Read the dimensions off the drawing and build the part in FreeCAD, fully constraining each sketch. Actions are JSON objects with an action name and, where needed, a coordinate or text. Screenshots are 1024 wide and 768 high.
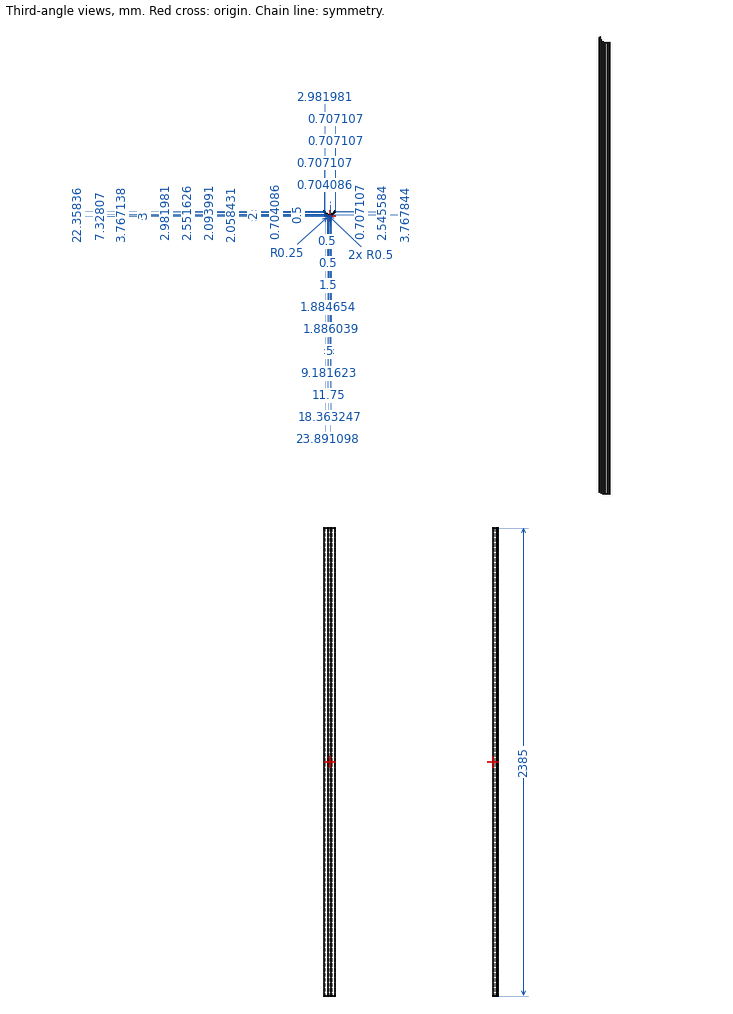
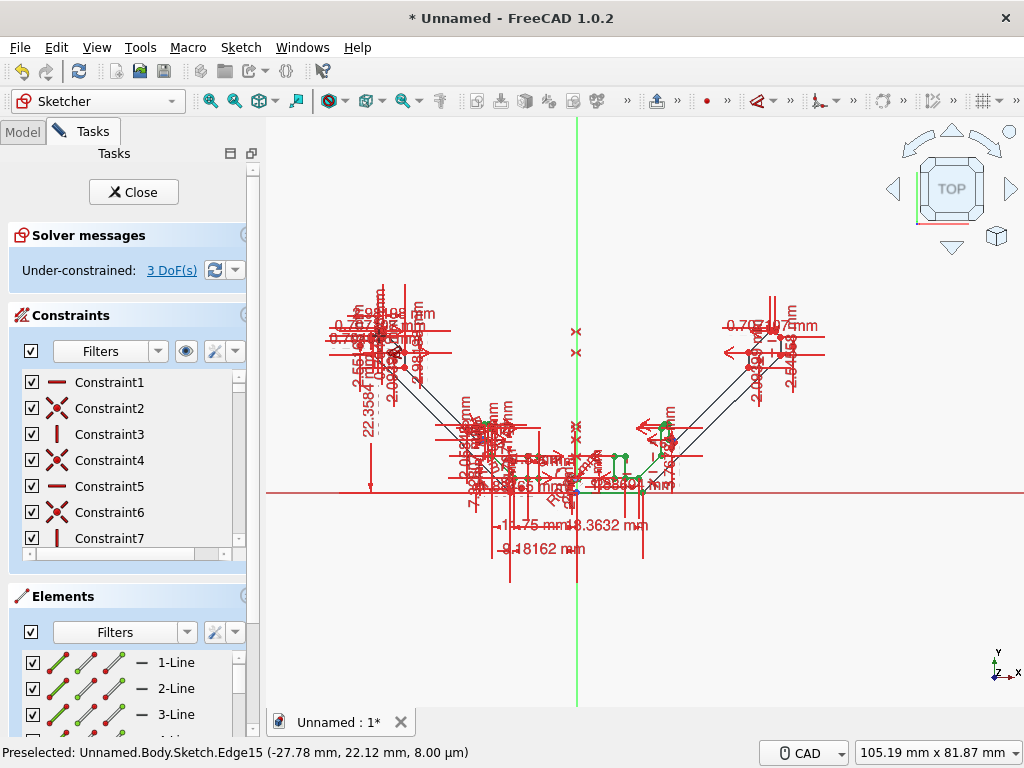
{"action": "scroll", "coordinate": [779, 335], "scroll_direction": "up", "scroll_amount": 11}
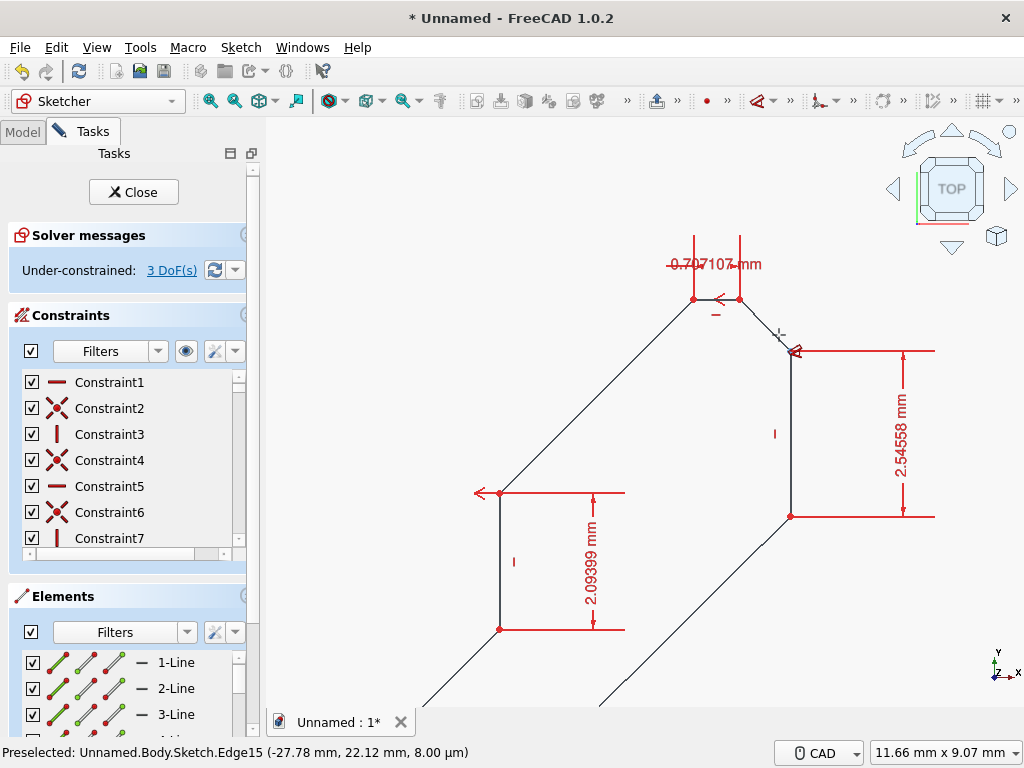
{"action": "left_click", "coordinate": [775, 336]}
{"action": "left_click", "coordinate": [765, 385]}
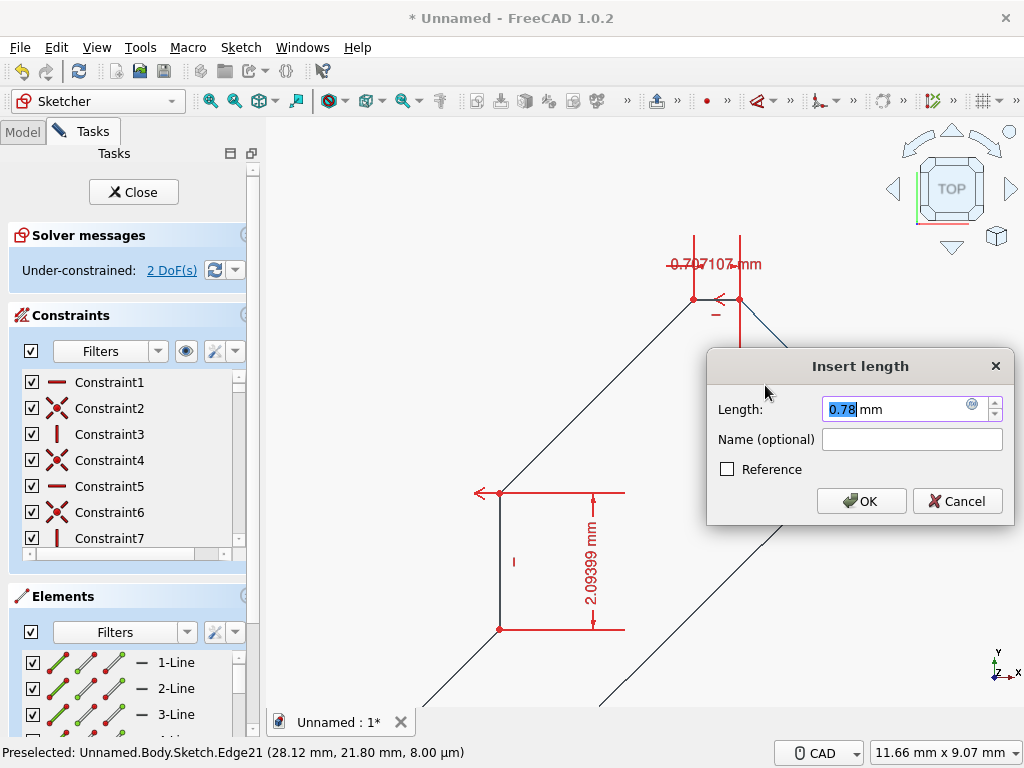
{"action": "type", "text": "0.707107"}
{"action": "key", "text": "Return"}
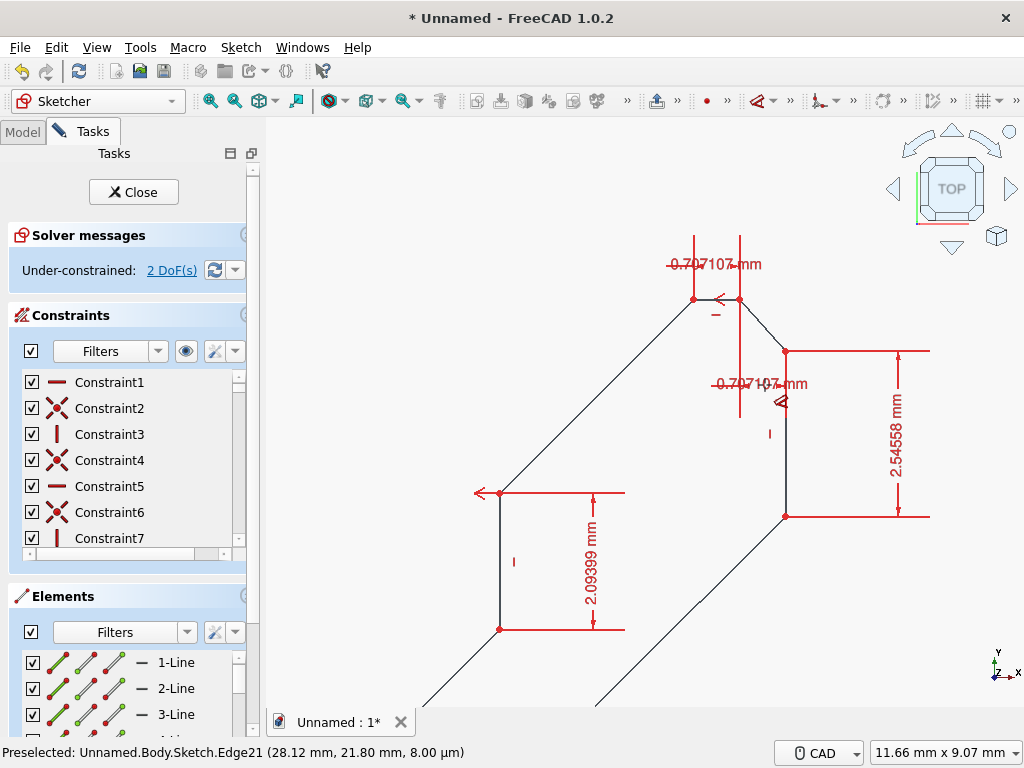
{"action": "left_click", "coordinate": [772, 336]}
{"action": "left_click", "coordinate": [820, 325]}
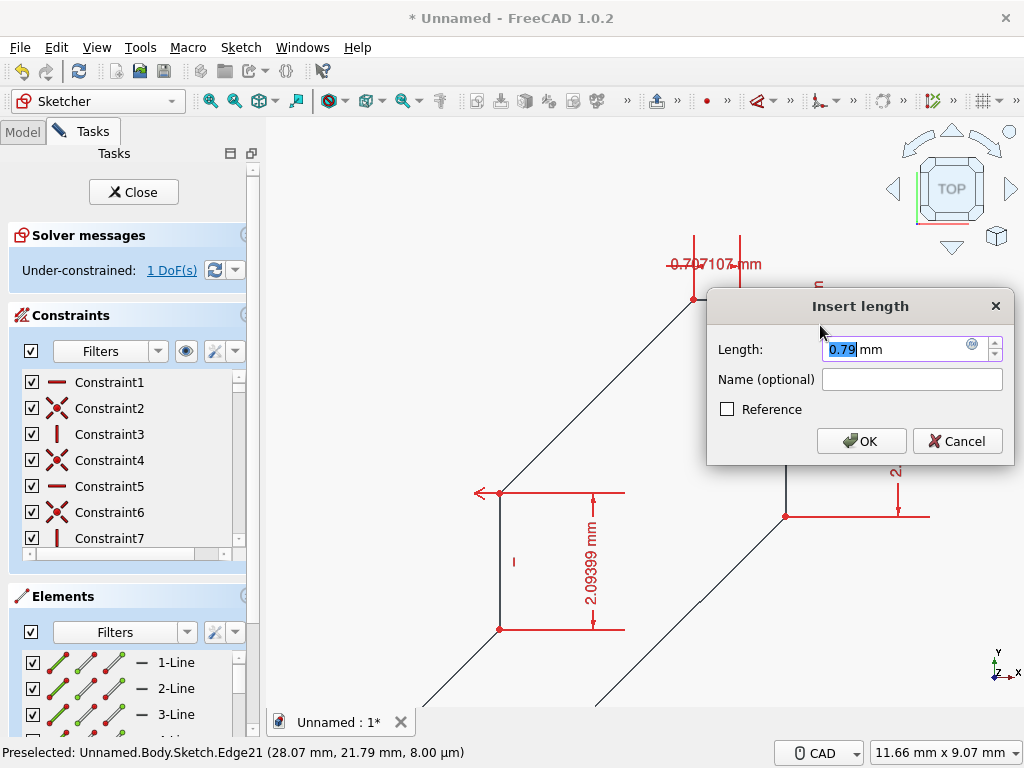
{"action": "type", "text": "0.707107"}
{"action": "key", "text": "Return"}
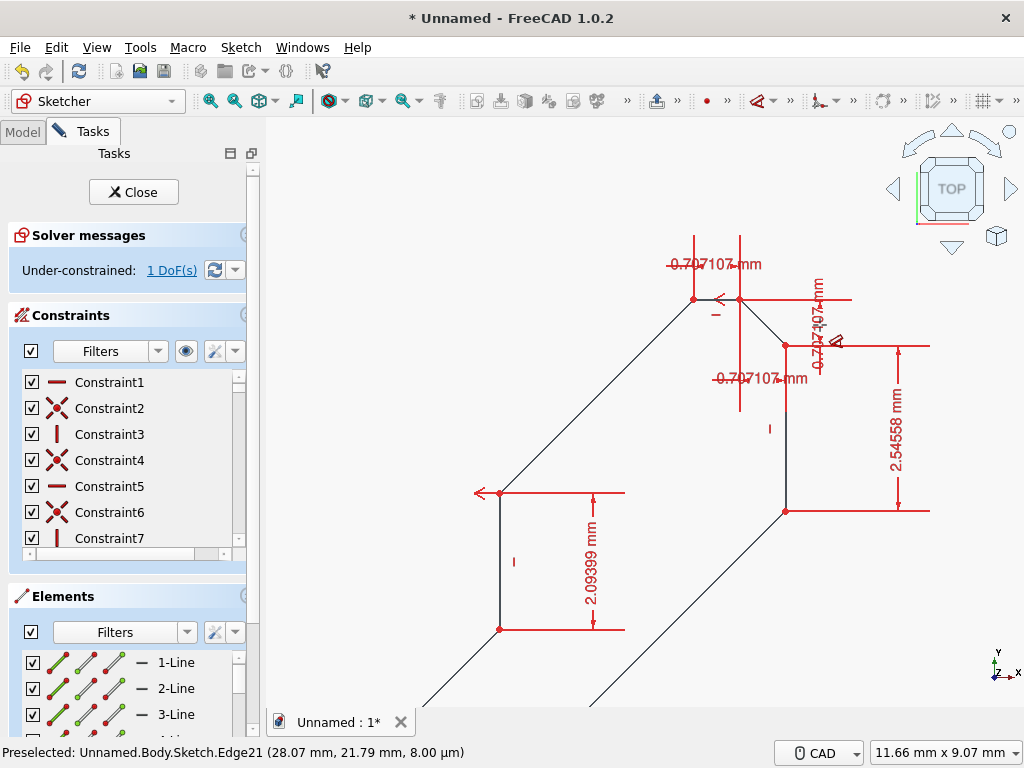
{"action": "scroll", "coordinate": [780, 335], "scroll_direction": "down", "scroll_amount": 11}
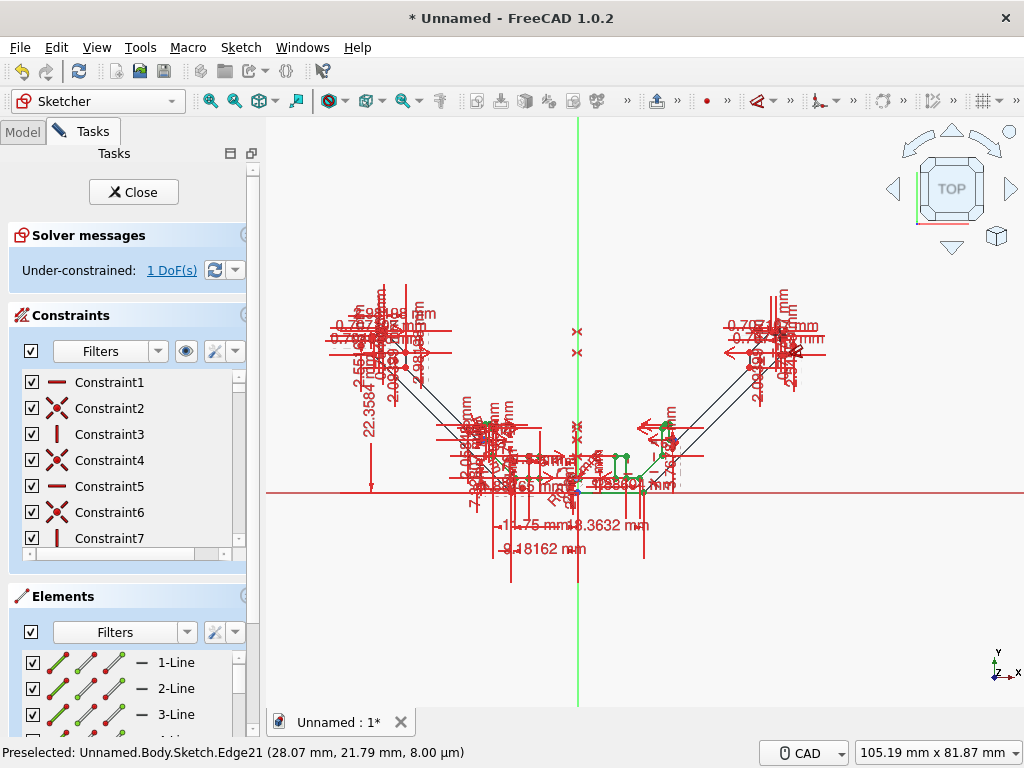
{"action": "left_click", "coordinate": [406, 368]}
{"action": "left_click", "coordinate": [452, 527]}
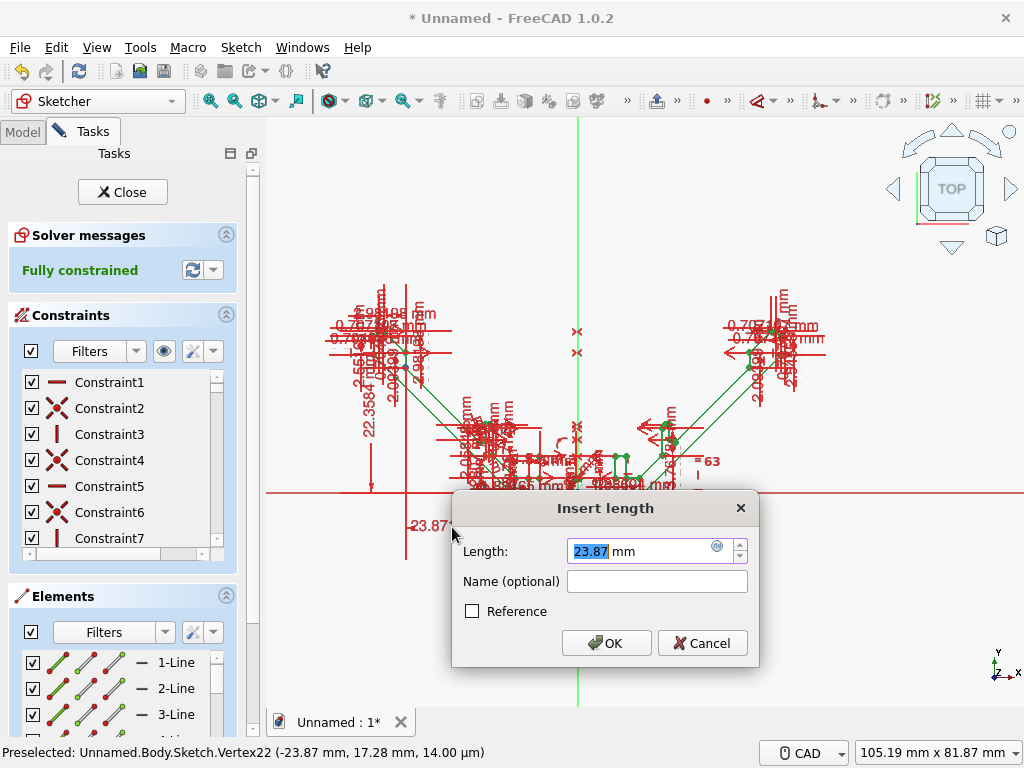
{"action": "type", "text": "23.891098"}
{"action": "key", "text": "Return"}
{"action": "key", "text": "Escape"}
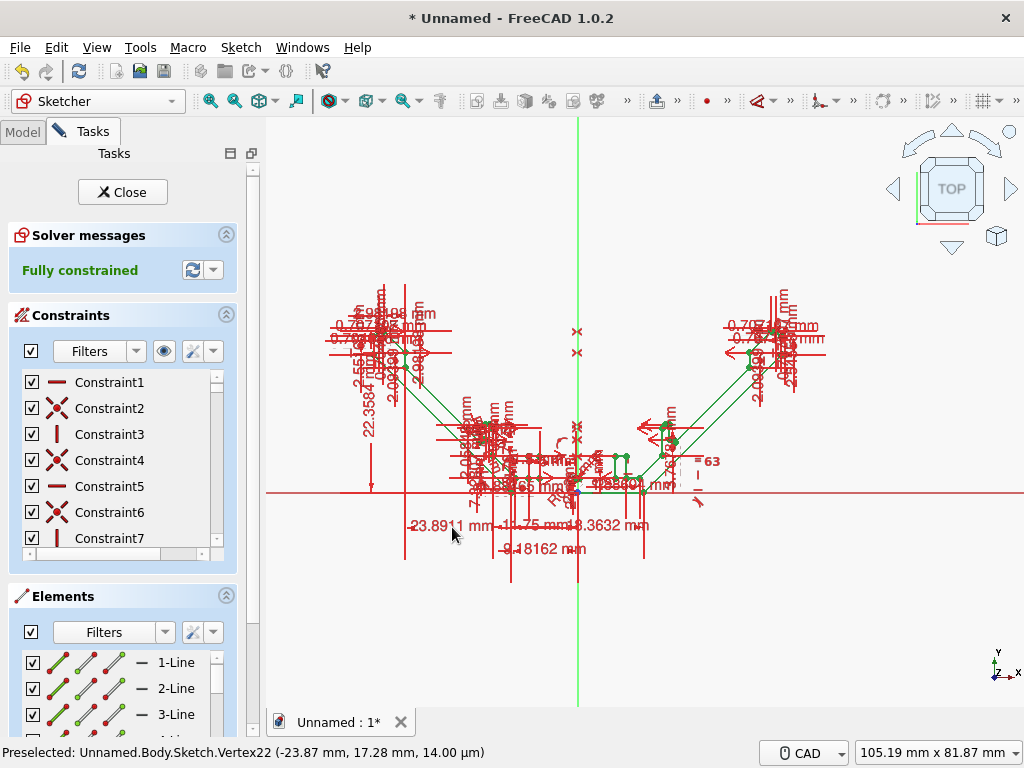
{"action": "left_click", "coordinate": [123, 192]}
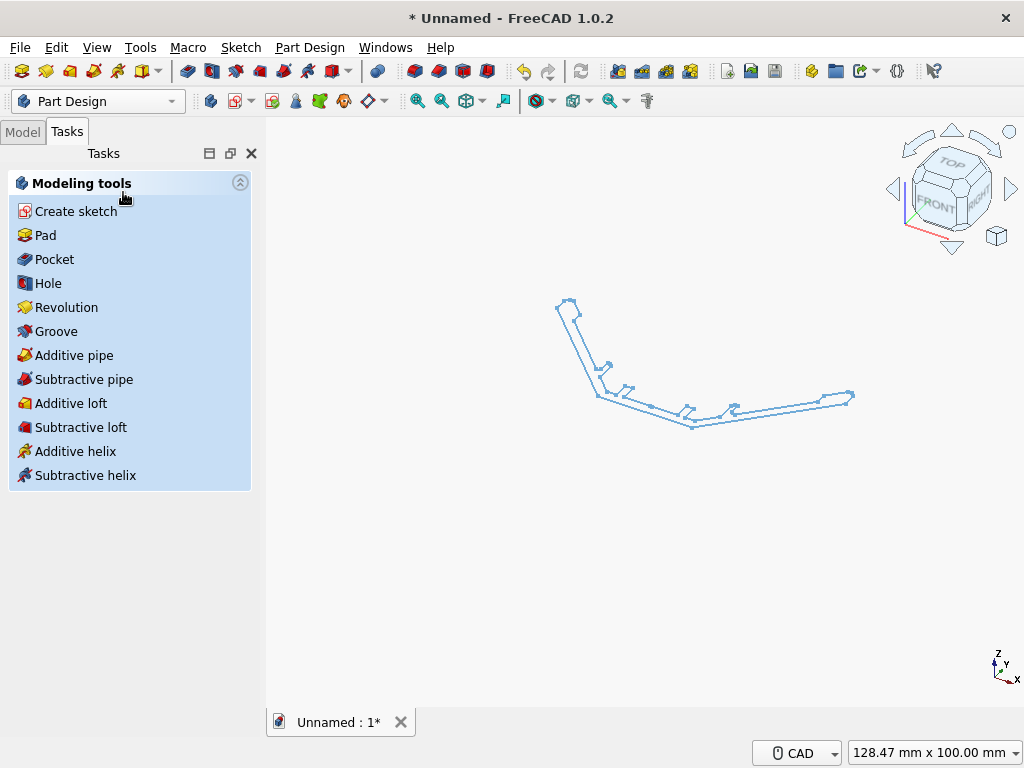
{"action": "left_click", "coordinate": [22, 72]}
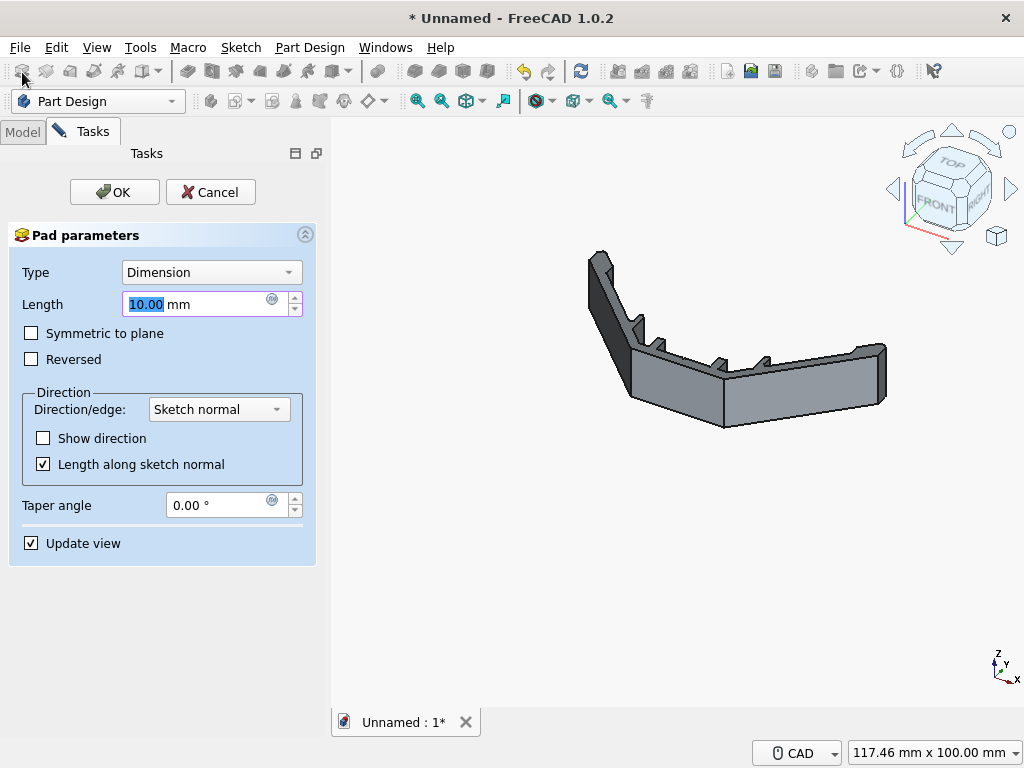
{"action": "type", "text": "2385"}
{"action": "key", "text": "Tab"}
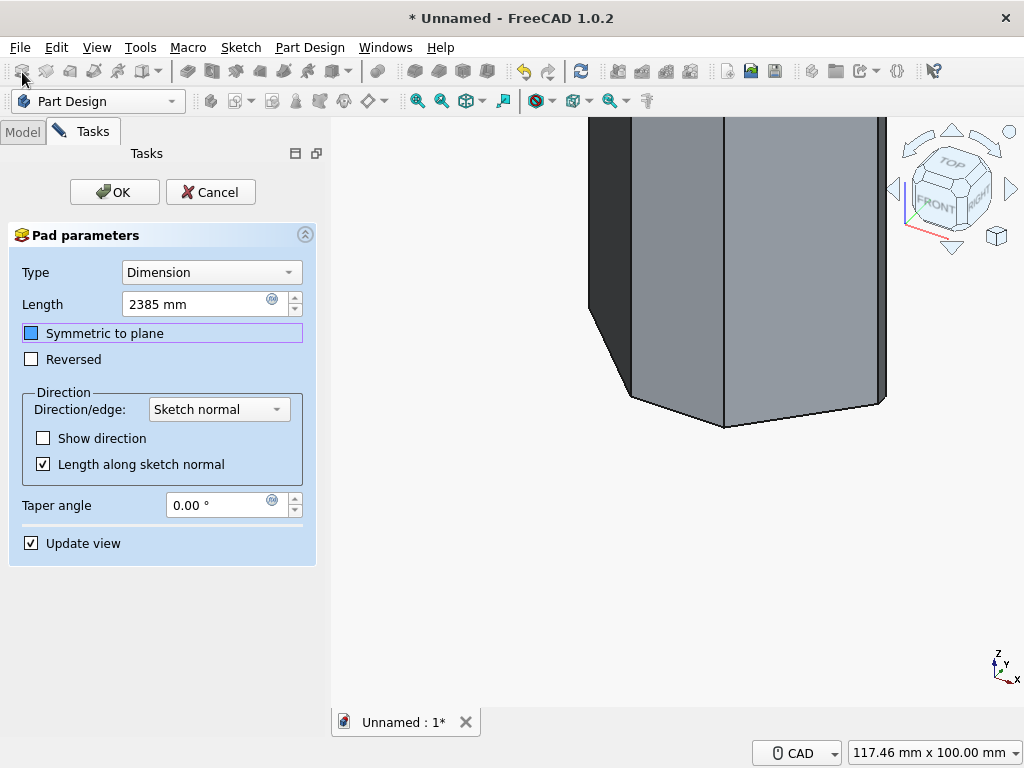
{"action": "left_click", "coordinate": [30, 333]}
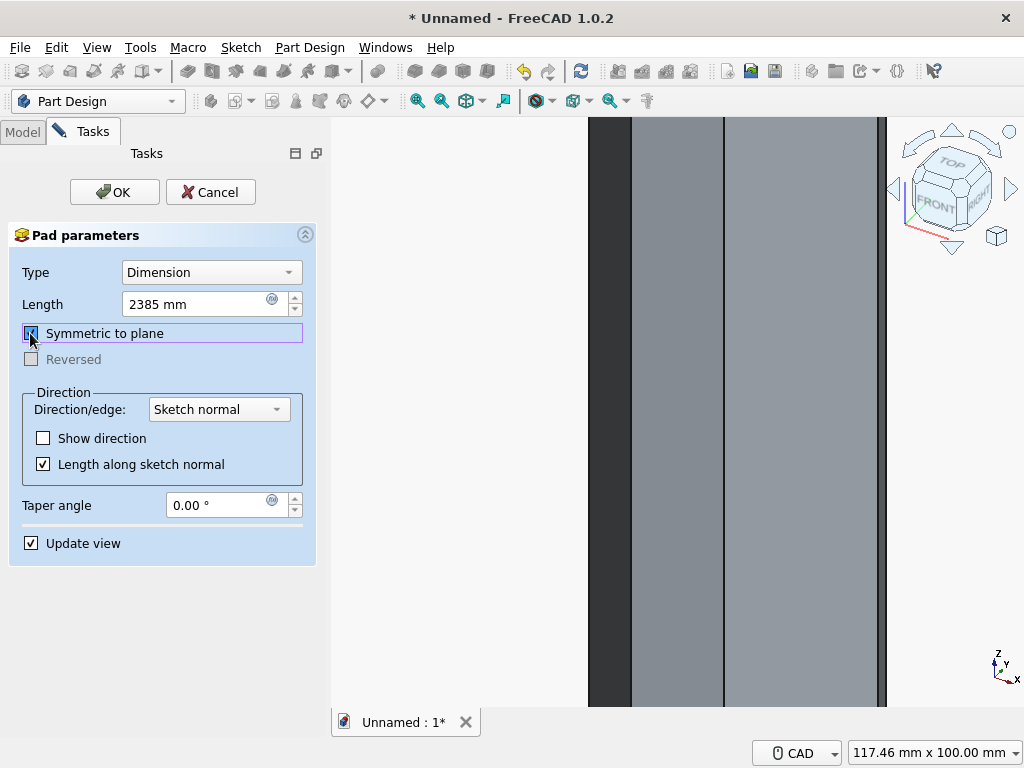
{"action": "left_click", "coordinate": [115, 192]}